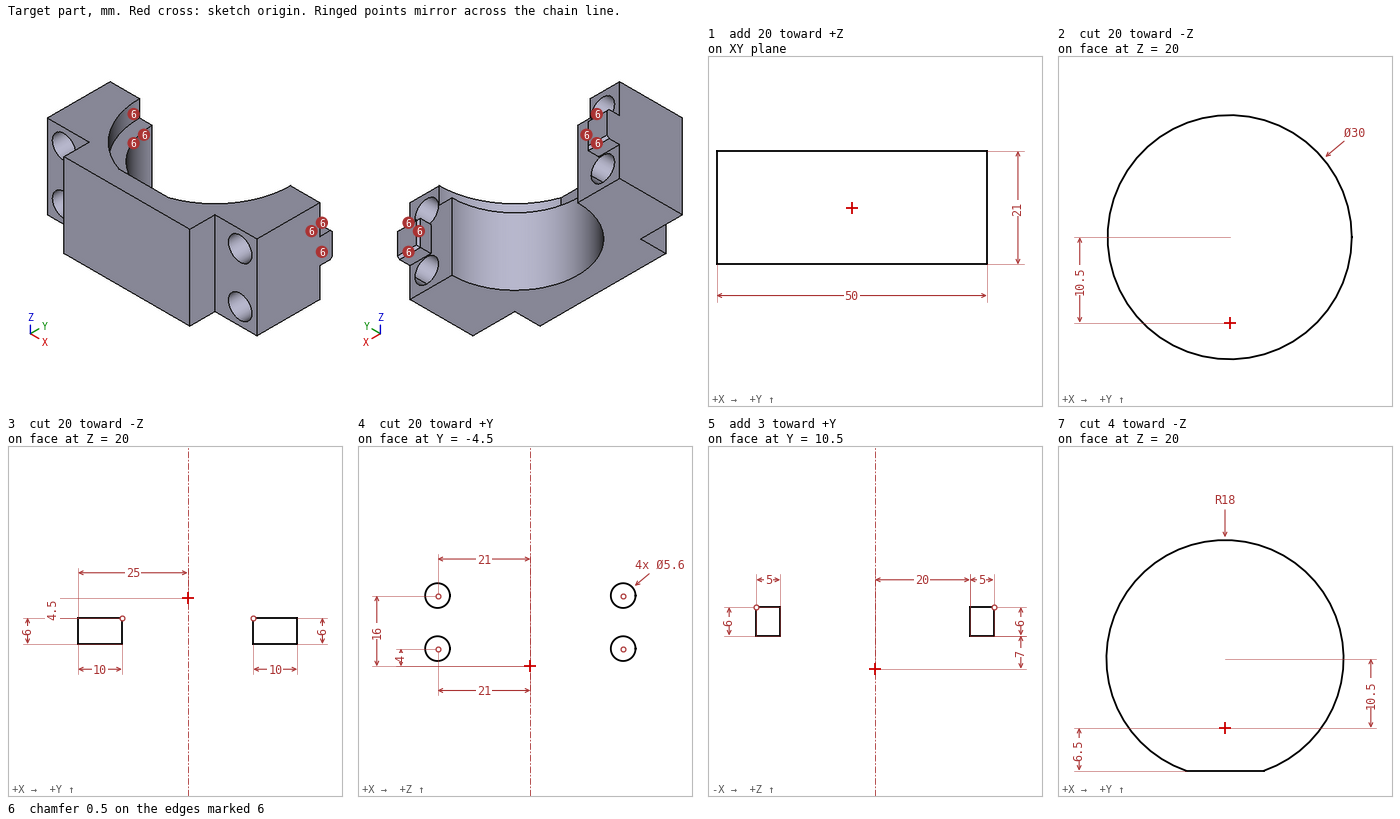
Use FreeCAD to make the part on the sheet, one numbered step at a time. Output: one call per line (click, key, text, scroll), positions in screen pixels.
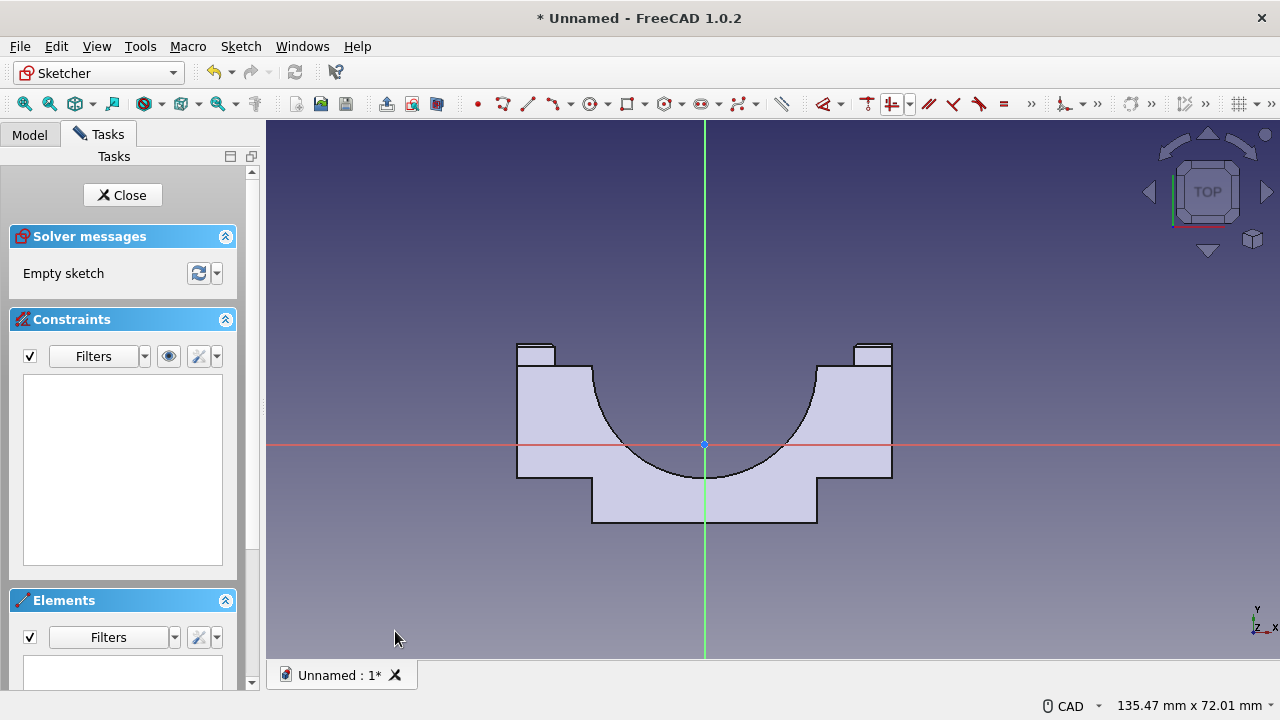
key(g)
key(l)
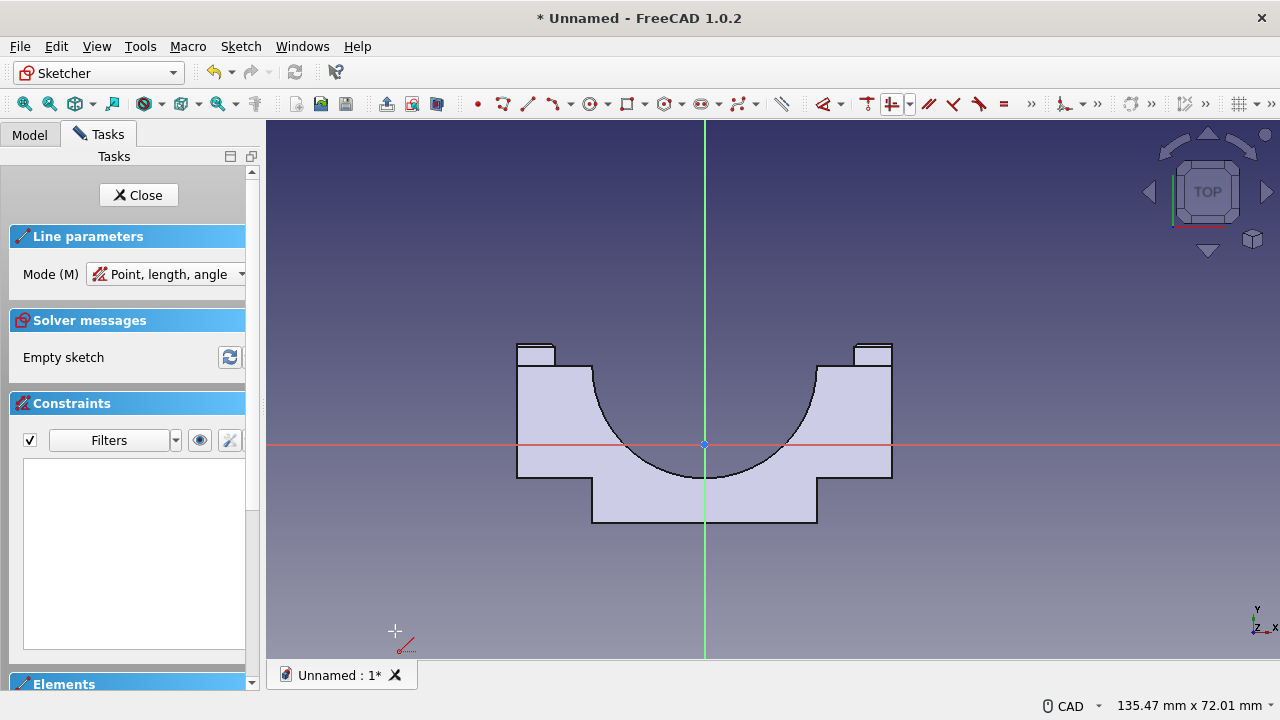
click(660, 493)
click(749, 493)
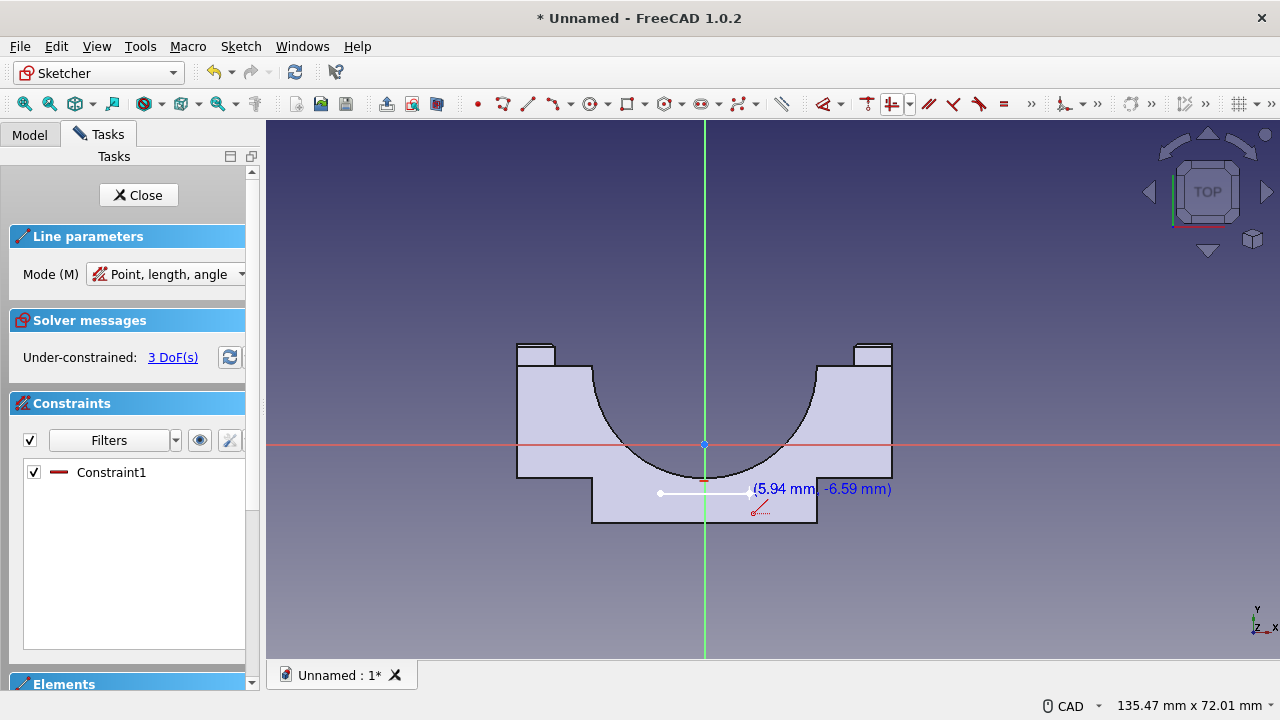
click(552, 104)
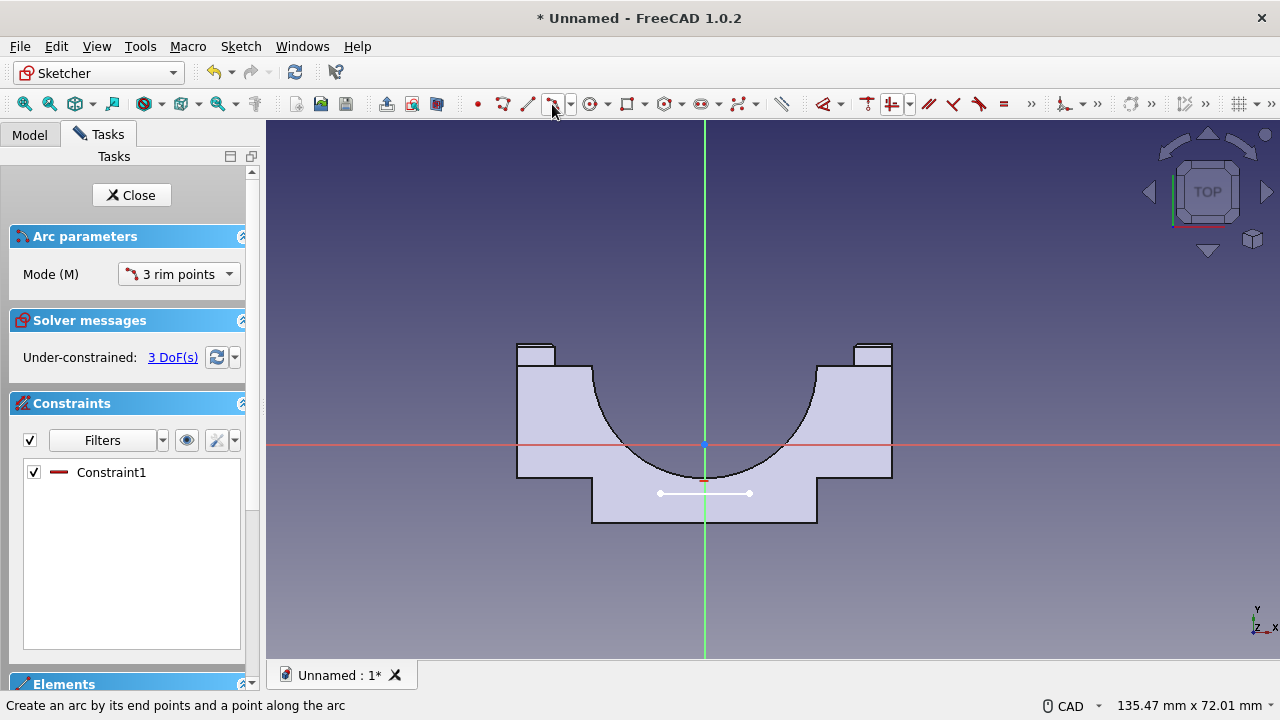
click(749, 494)
click(660, 494)
click(776, 252)
key(Escape)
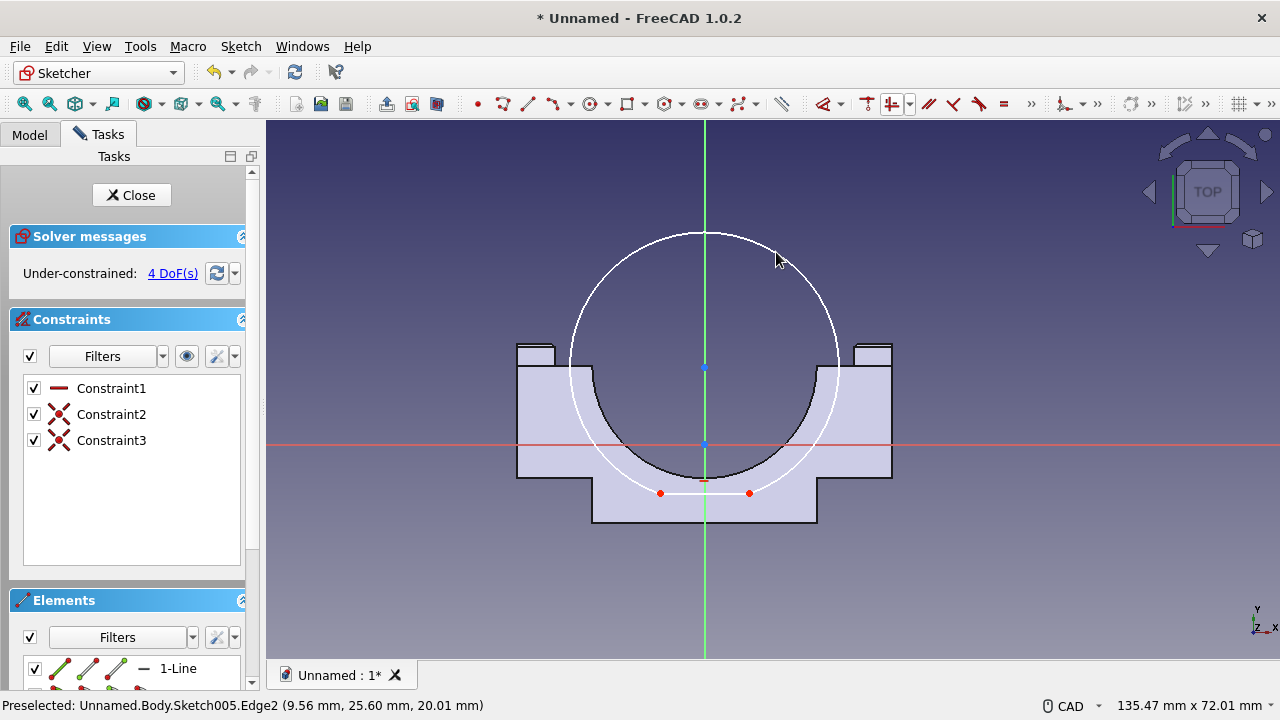
click(705, 367)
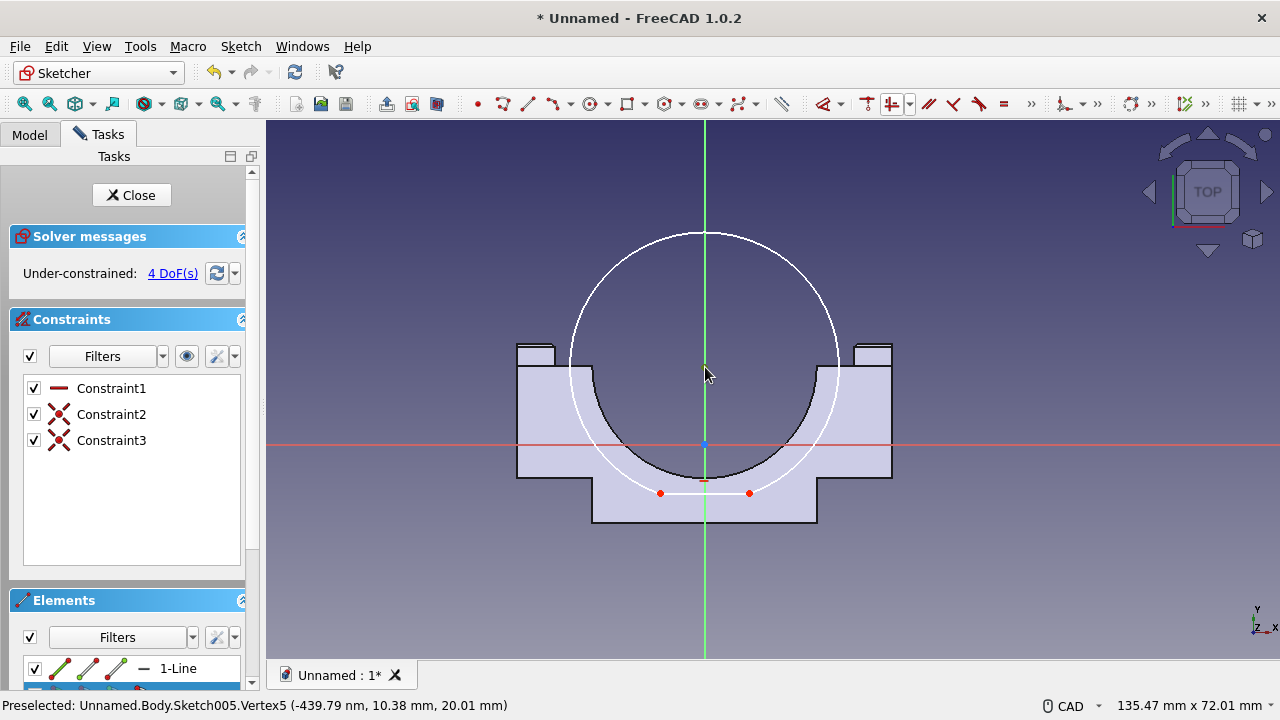
click(705, 596)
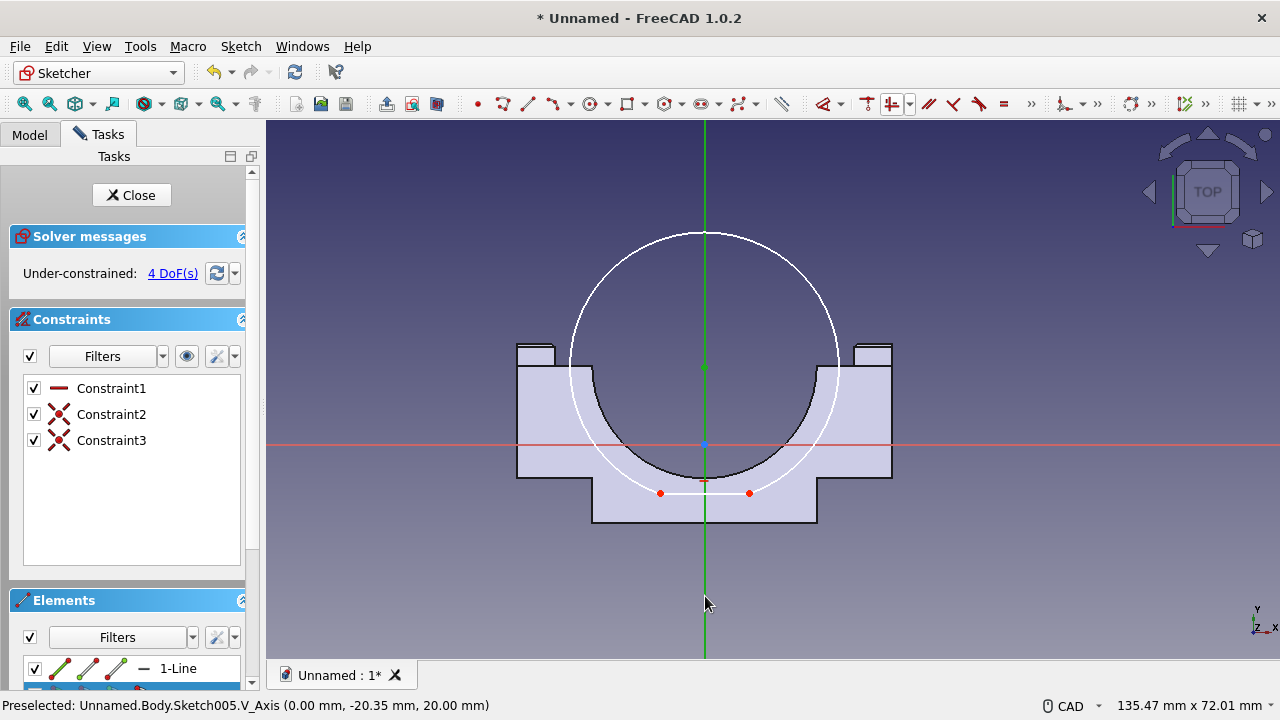
key(c)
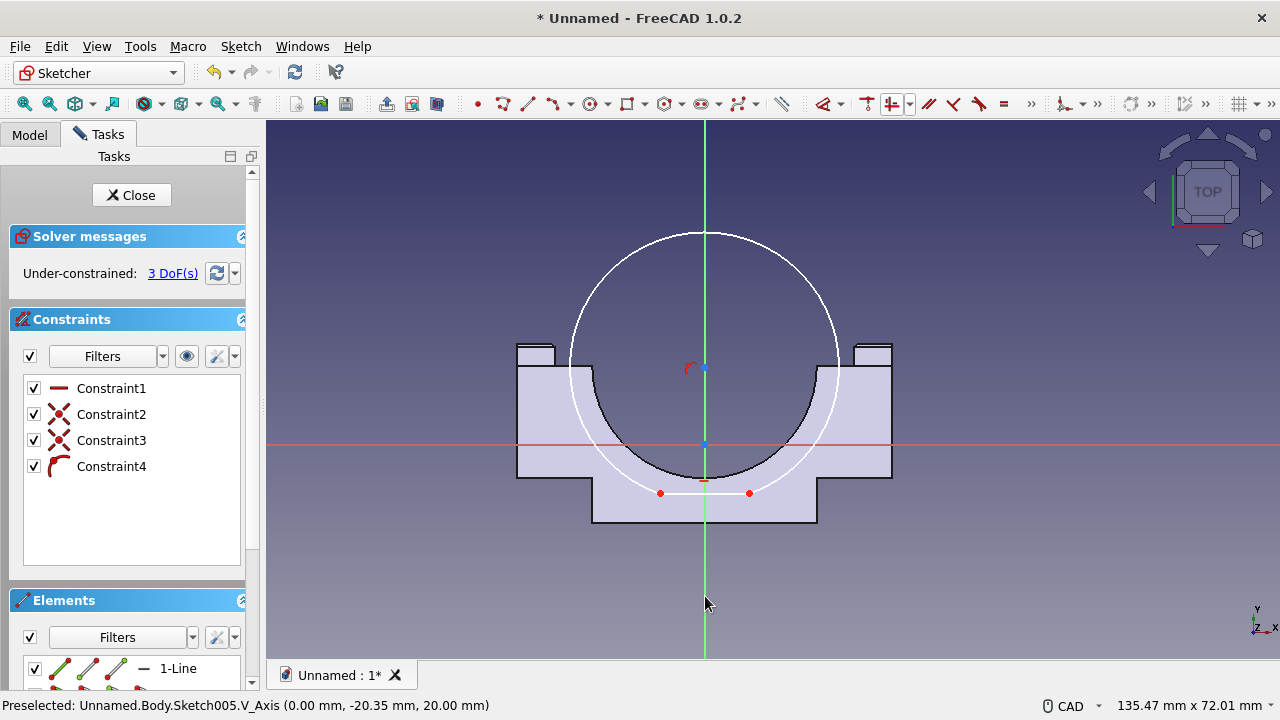
click(822, 104)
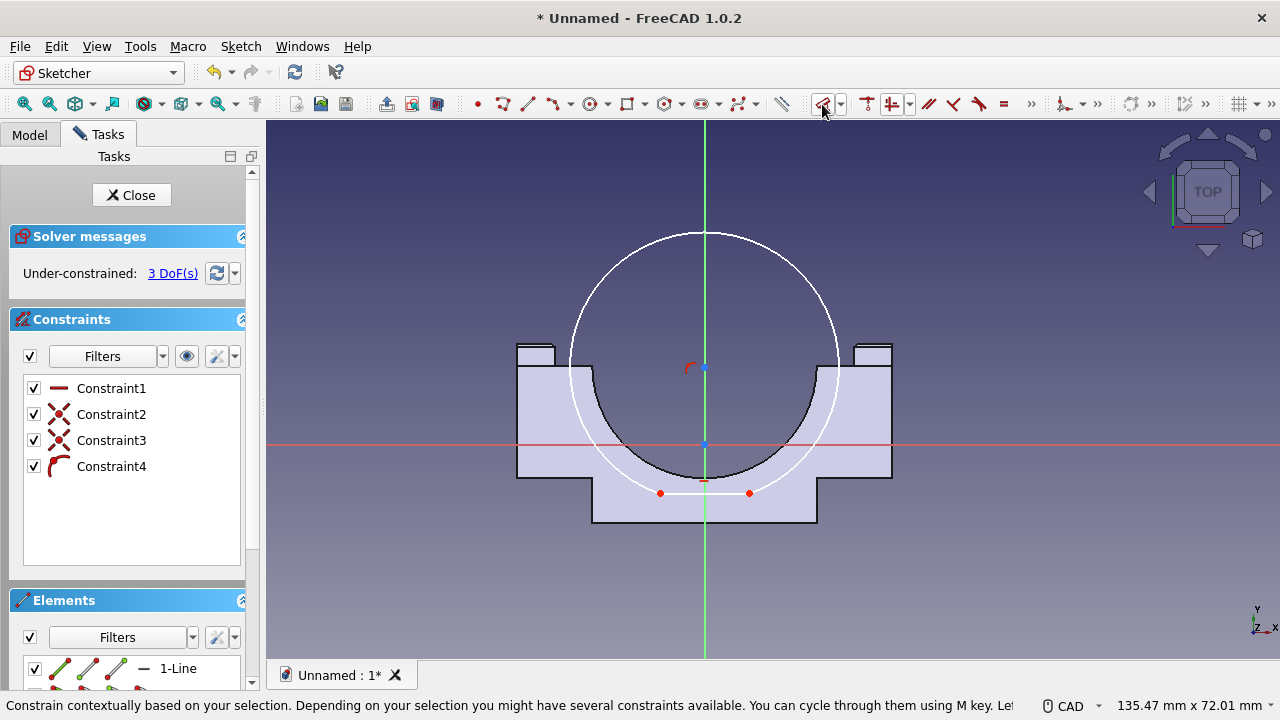
click(826, 309)
click(855, 295)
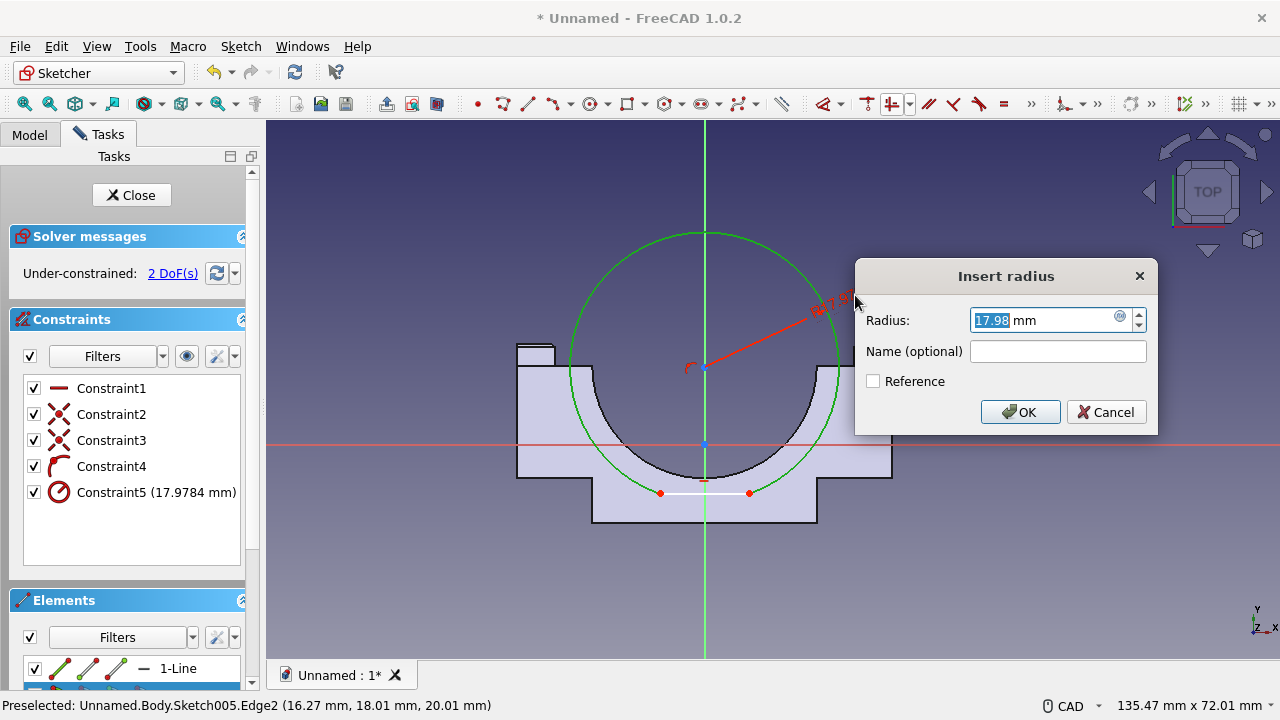
text(18)
key(Return)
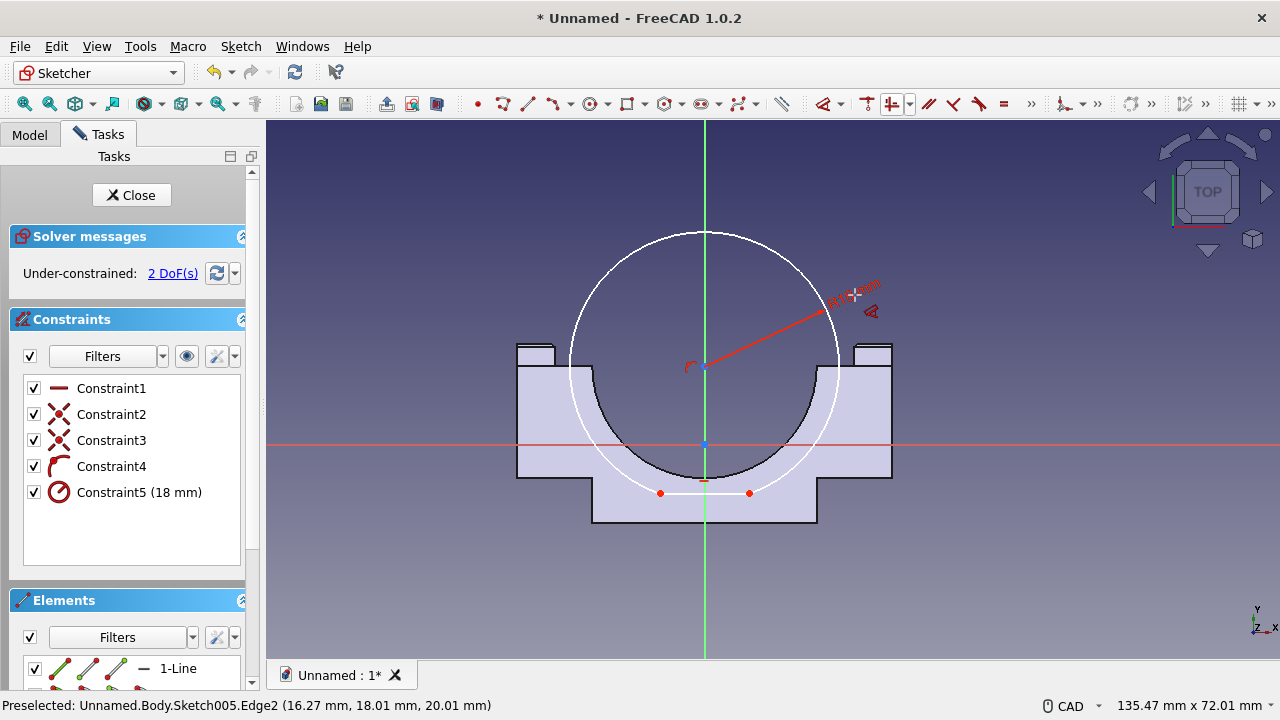
click(660, 494)
click(626, 458)